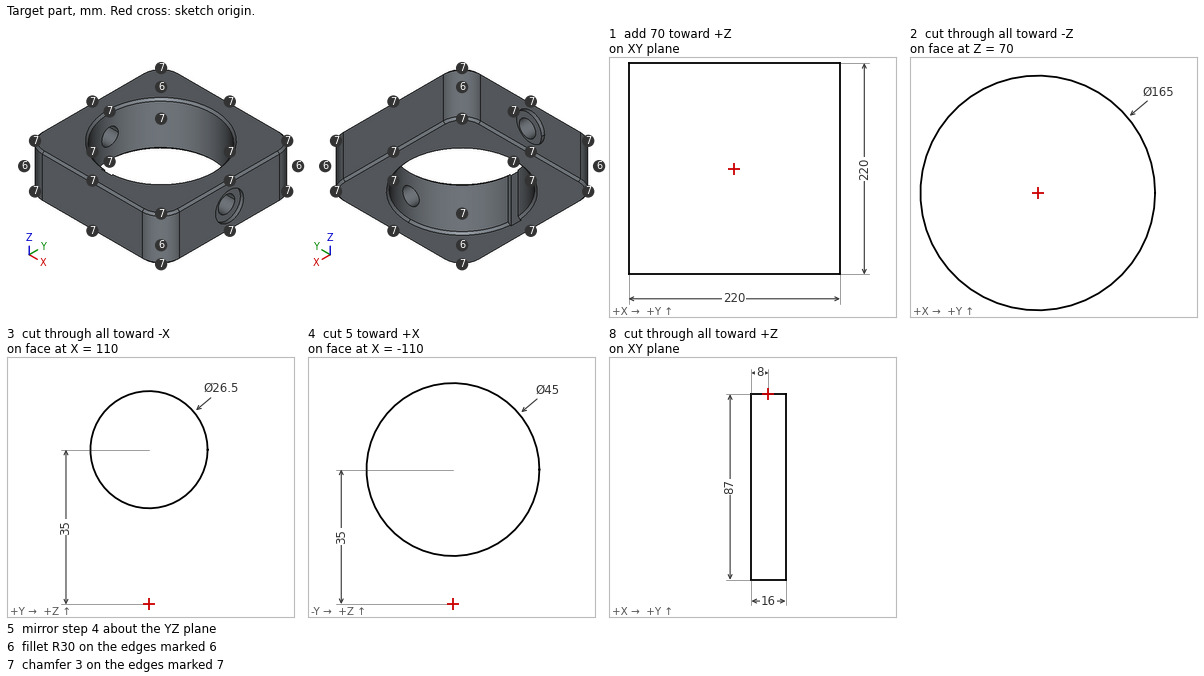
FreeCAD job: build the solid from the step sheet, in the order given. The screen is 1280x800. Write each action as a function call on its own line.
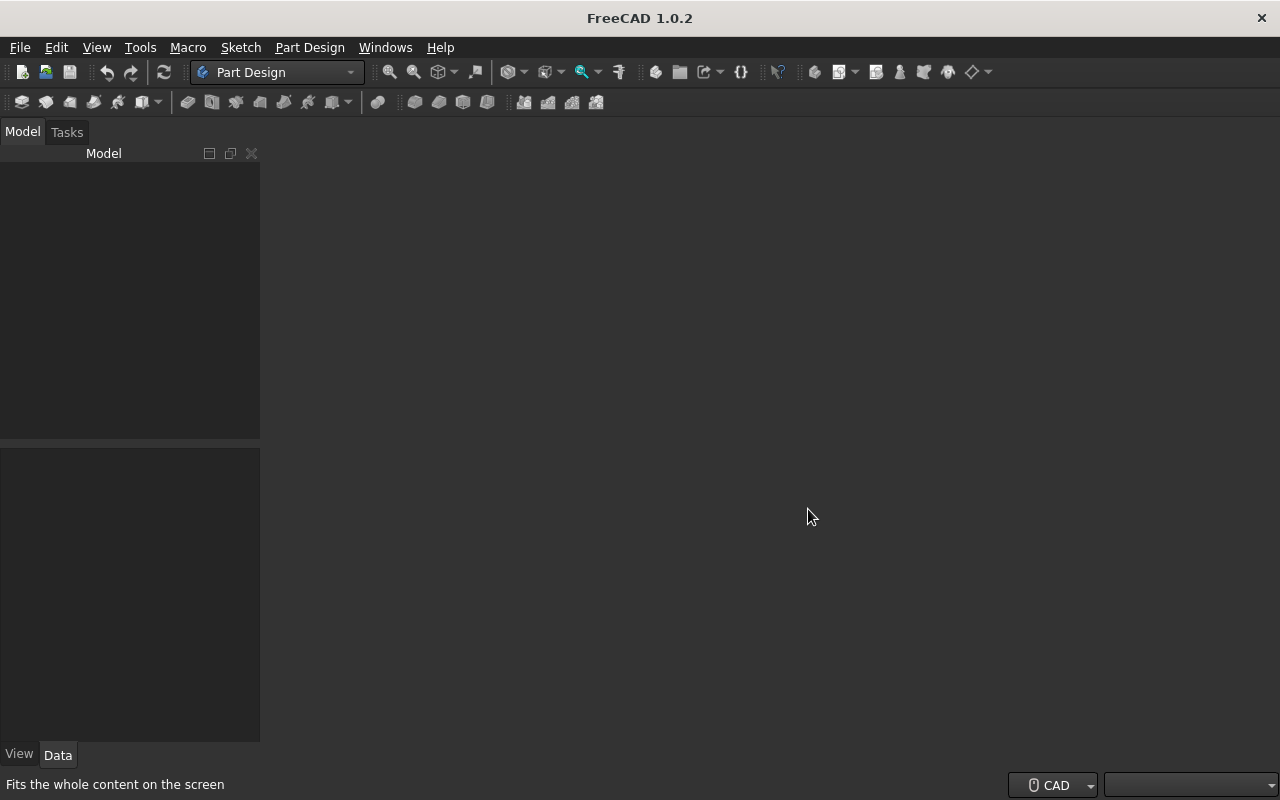
key(ctrl+n)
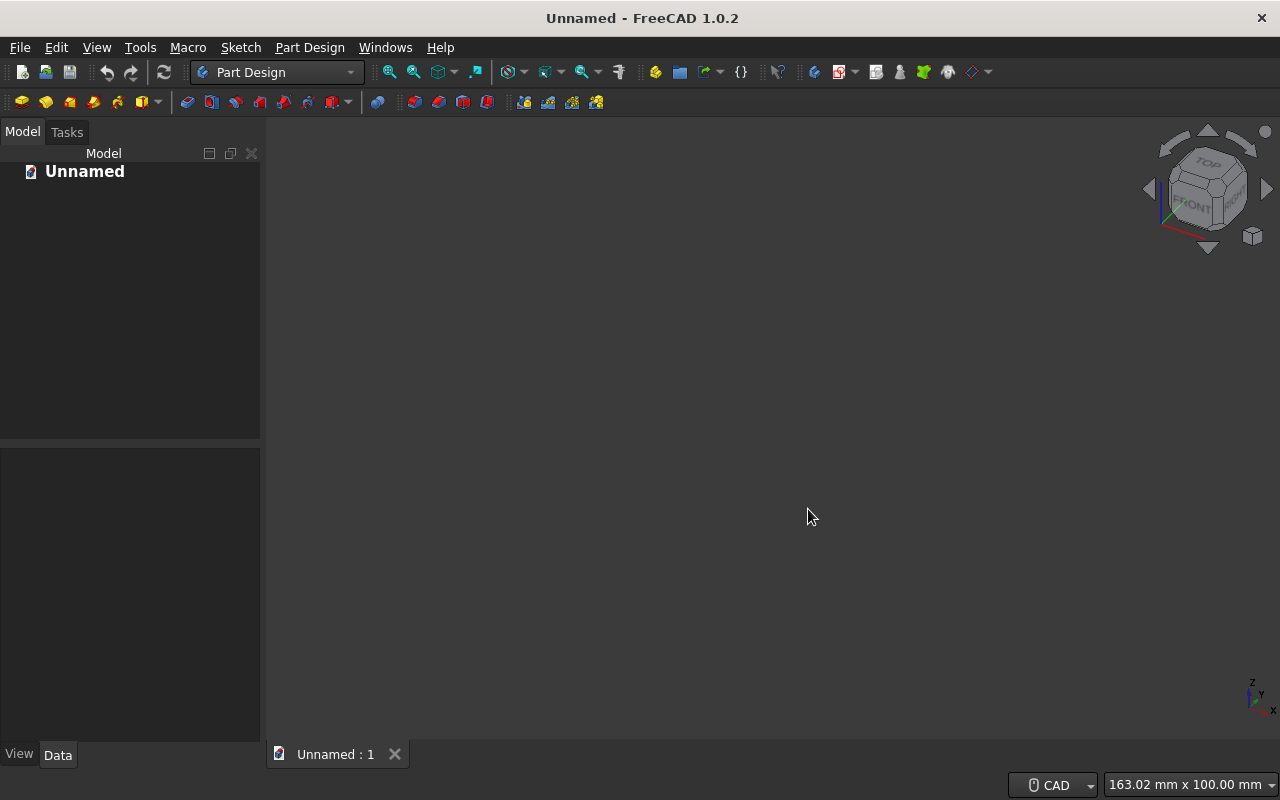
click(840, 72)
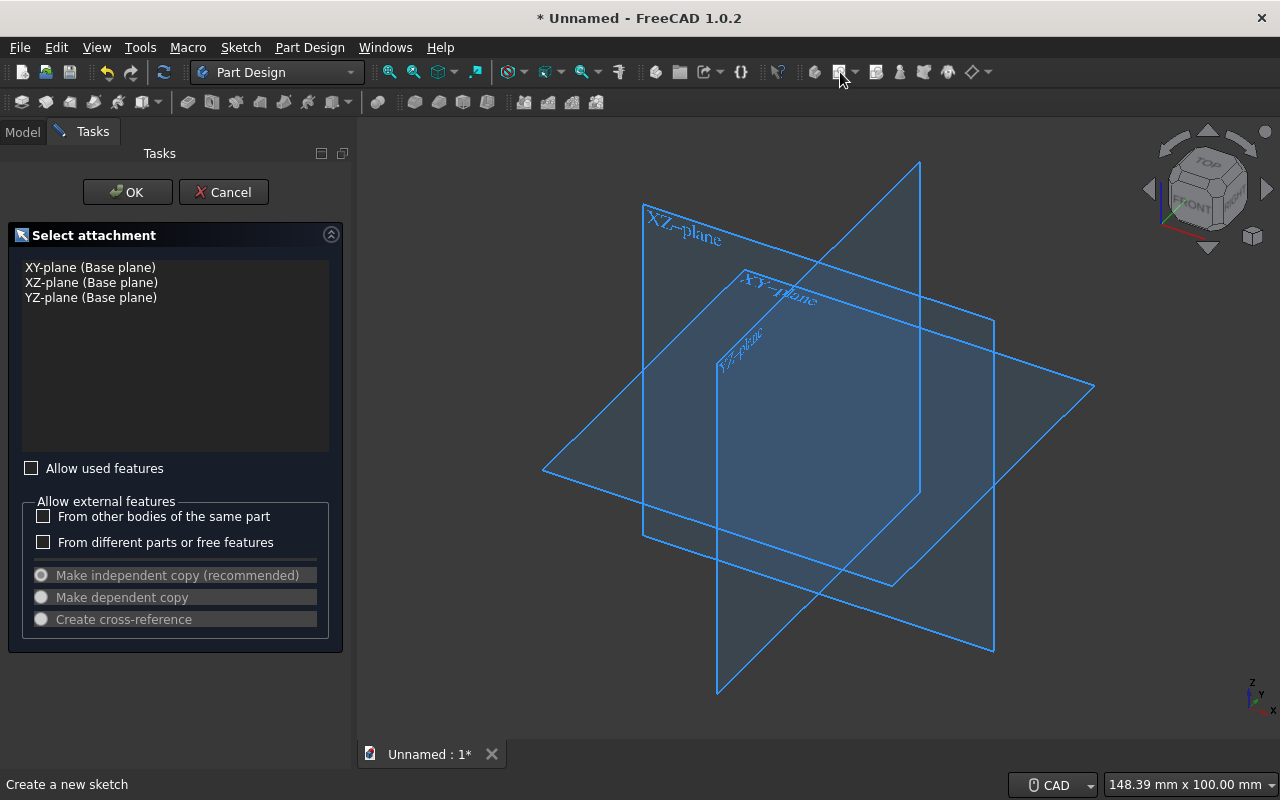
click(82, 268)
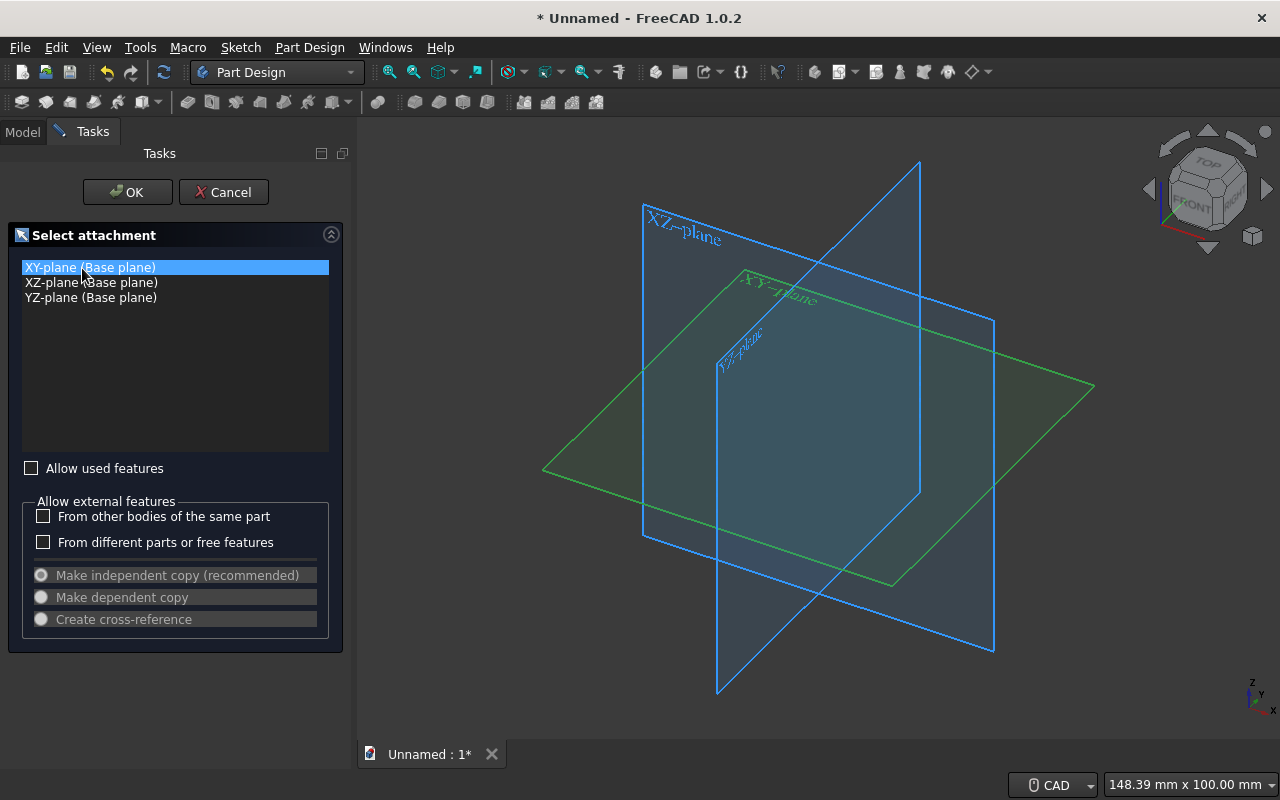
click(128, 192)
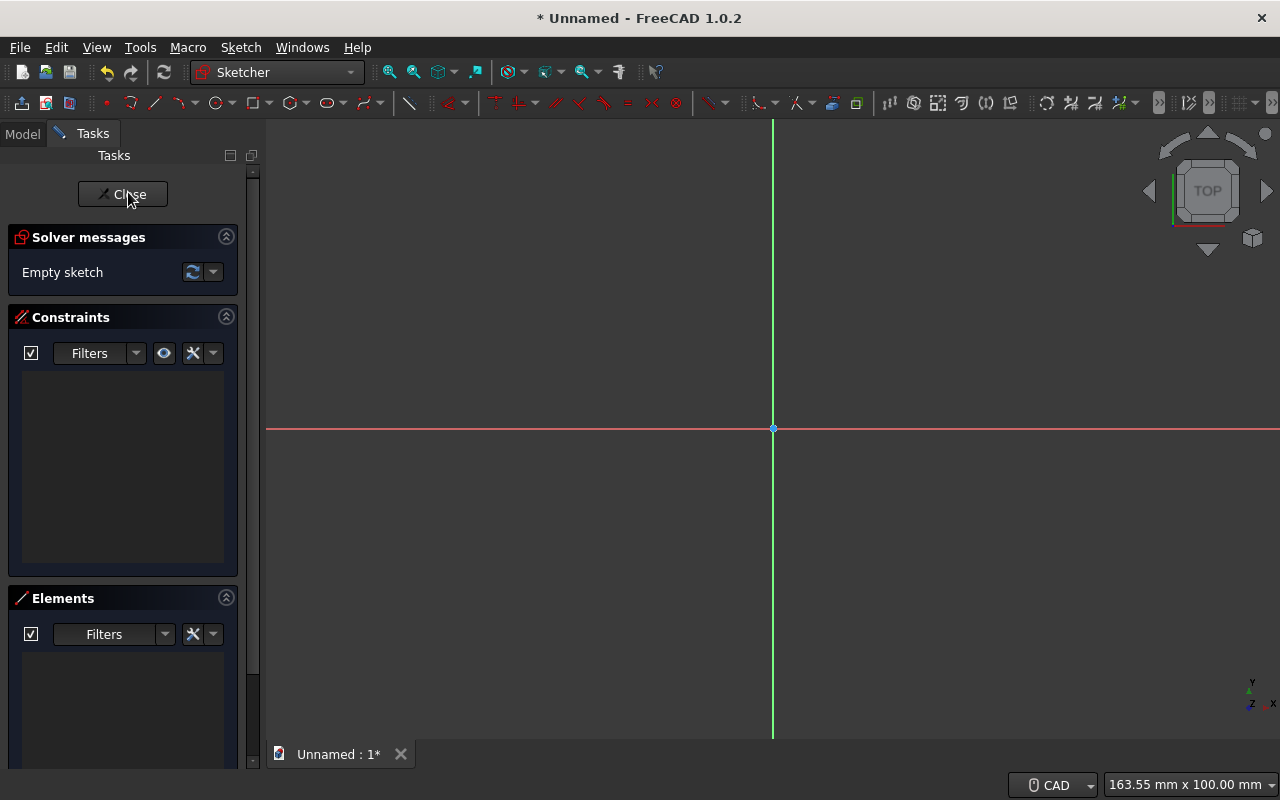
scroll(675, 429, down, 6)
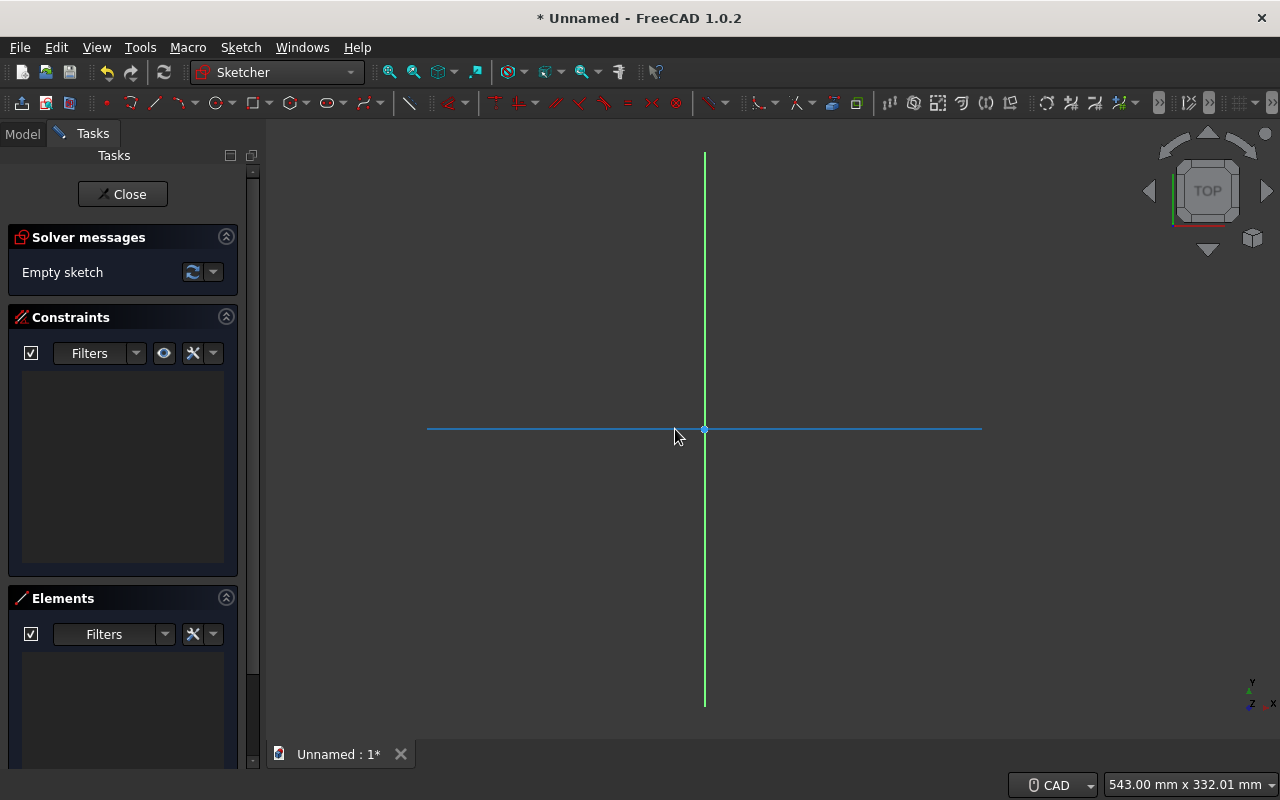
key(g)
key(v)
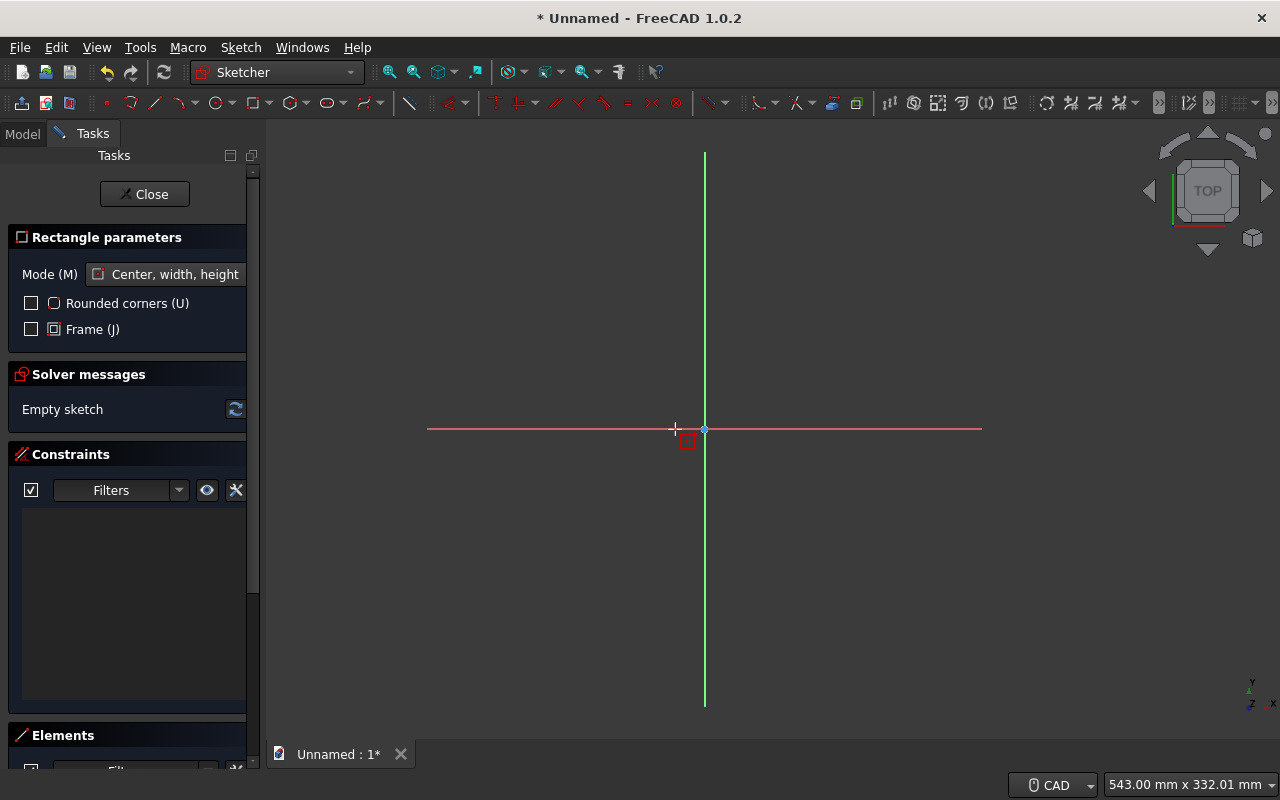
click(705, 429)
click(910, 224)
key(Escape)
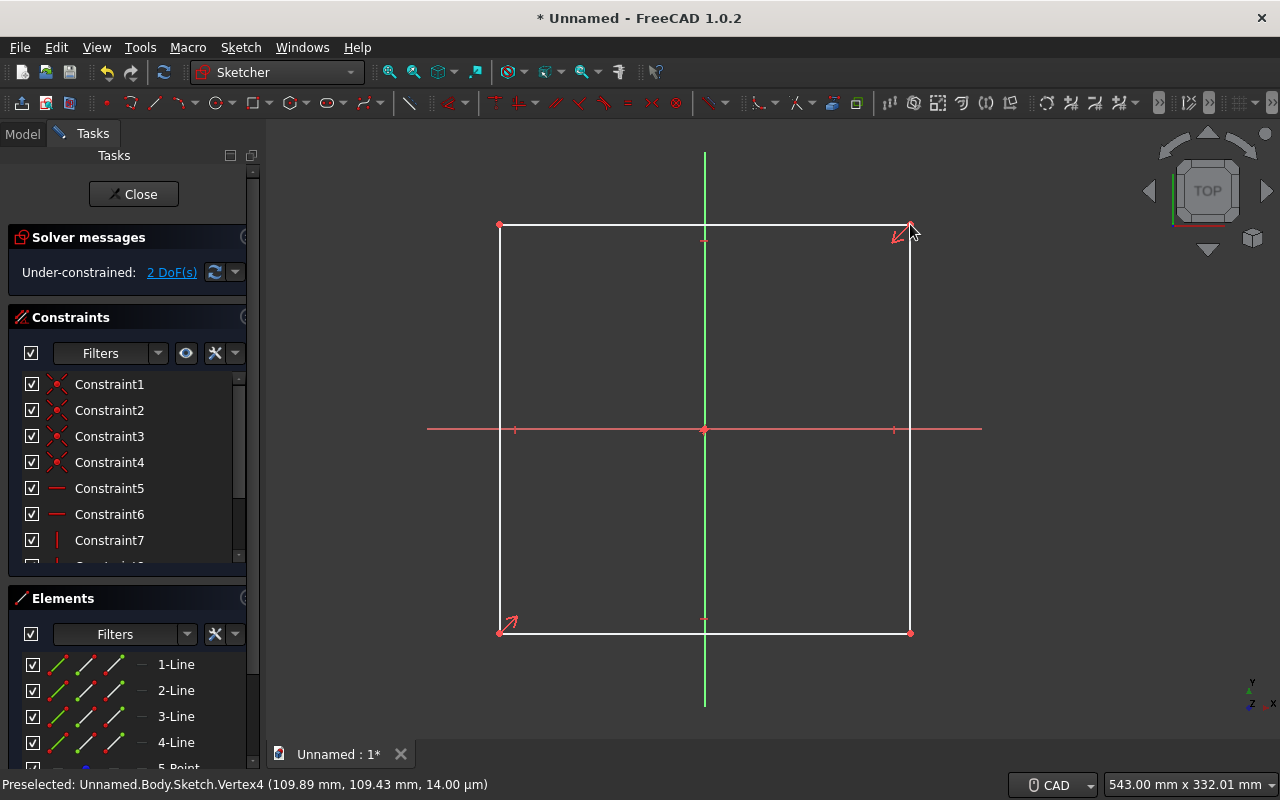
key(d)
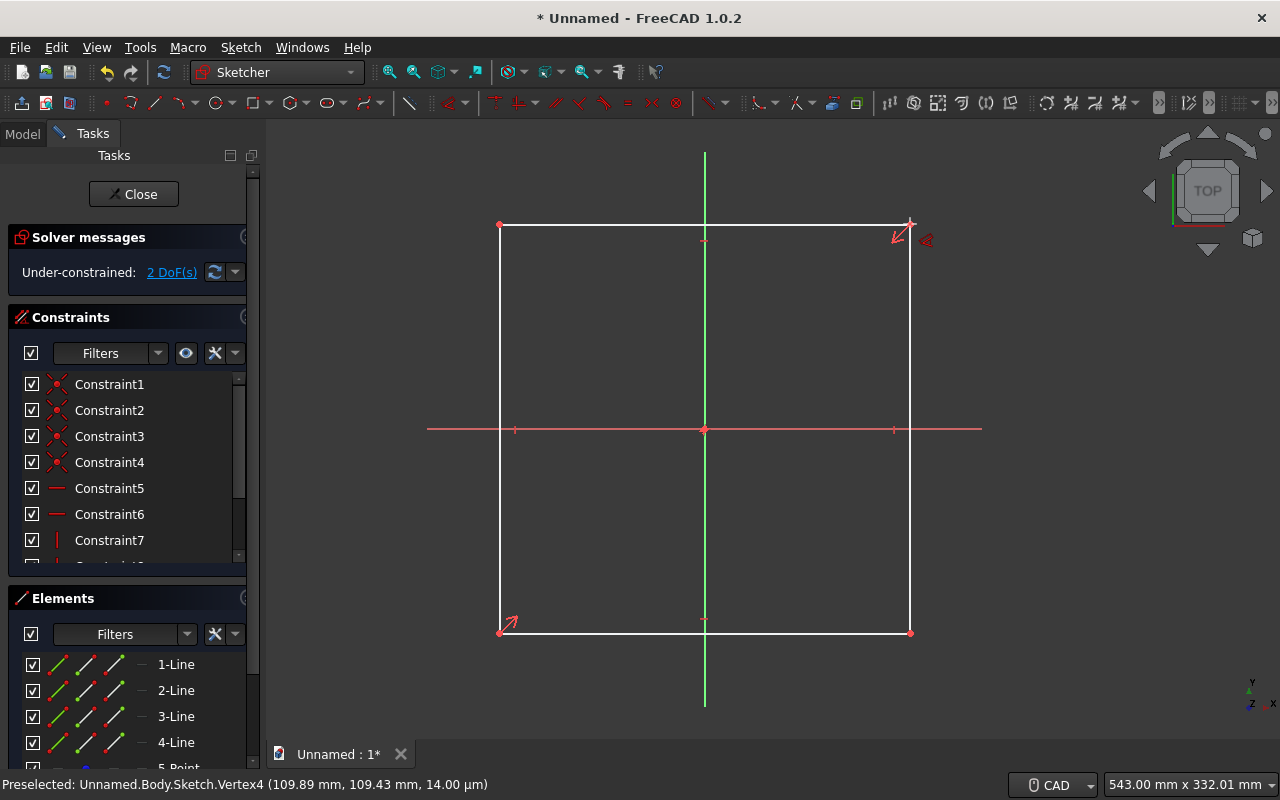
click(623, 634)
click(610, 668)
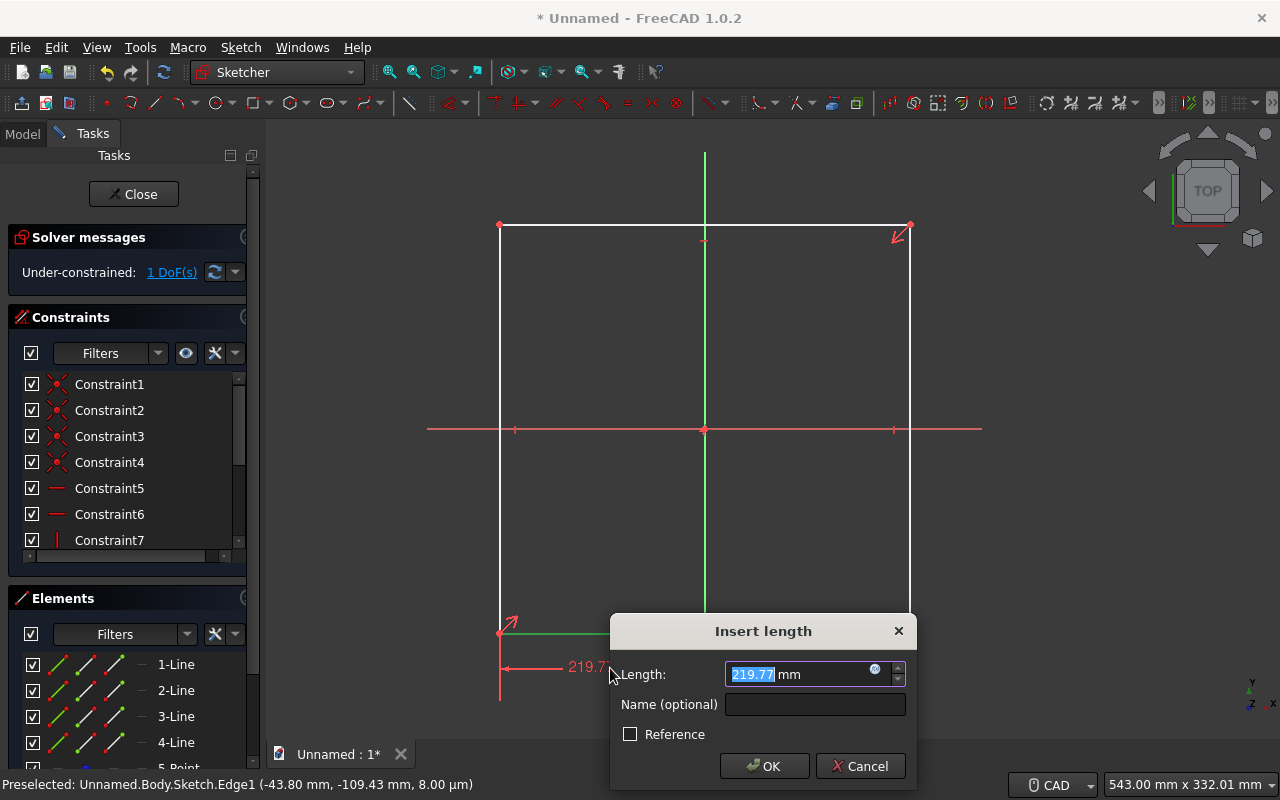
text(220)
key(Return)